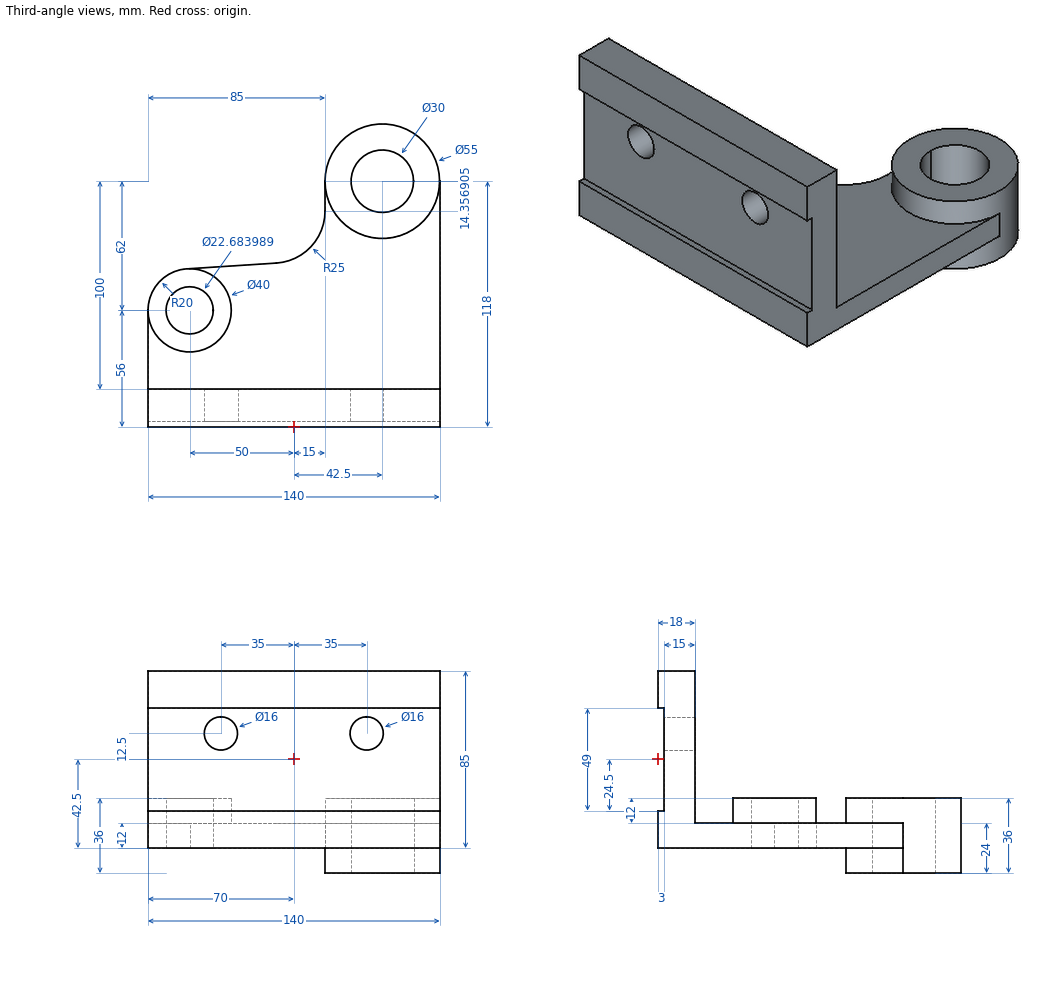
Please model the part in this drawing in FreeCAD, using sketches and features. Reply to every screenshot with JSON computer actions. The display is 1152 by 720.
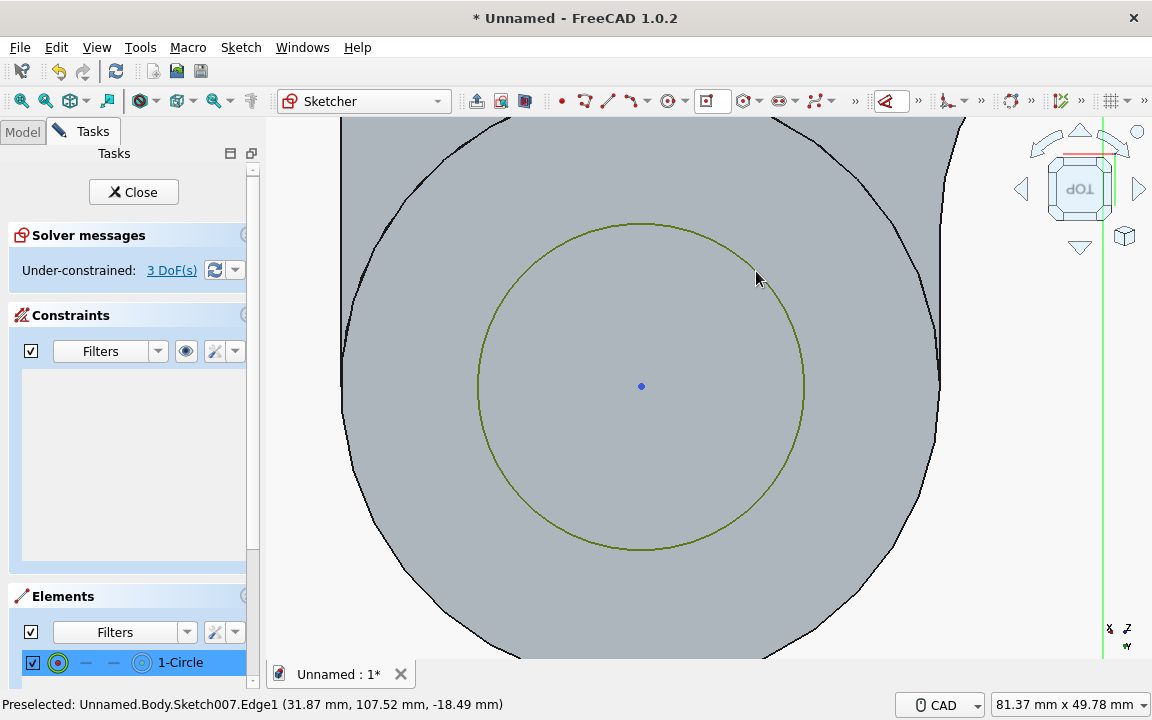
{"action": "left_click", "coordinate": [904, 102]}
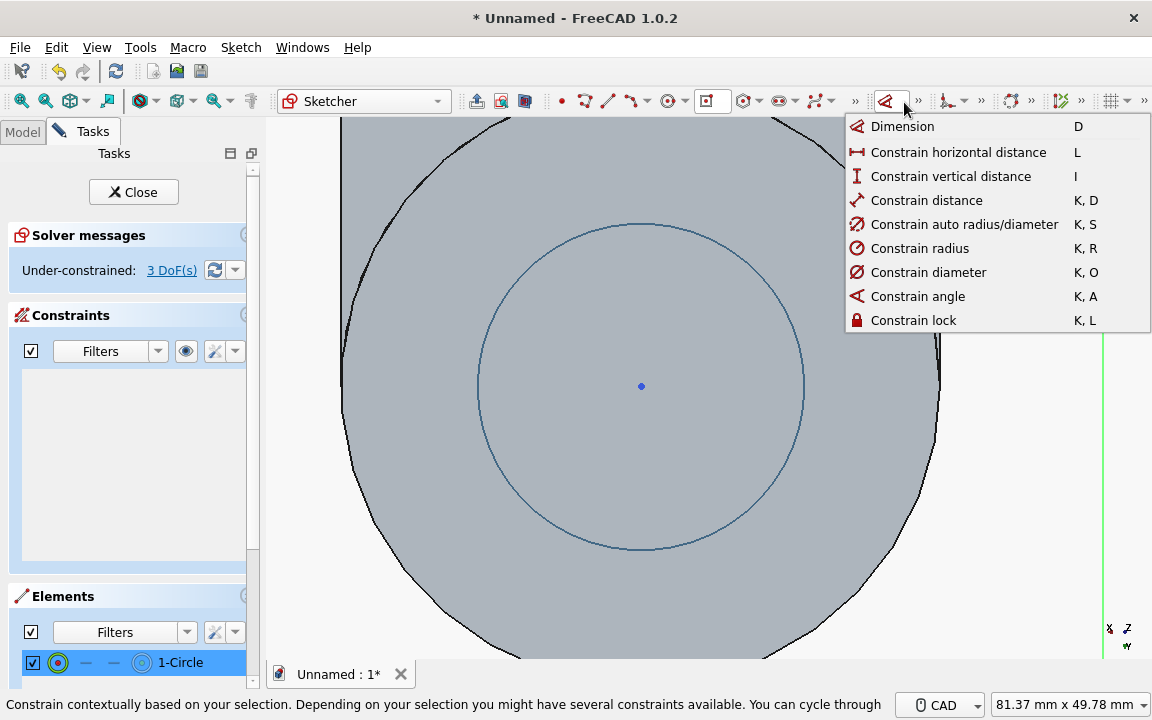
{"action": "left_click", "coordinate": [998, 272]}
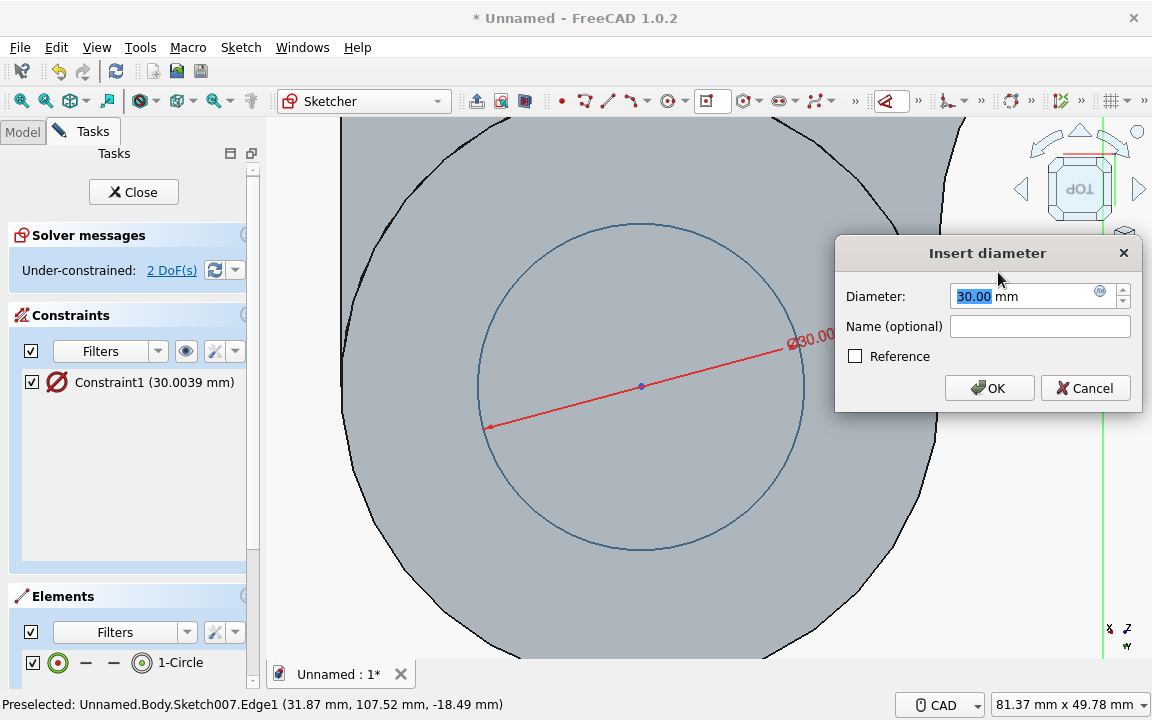
{"action": "type", "text": "30"}
{"action": "key", "text": "Return"}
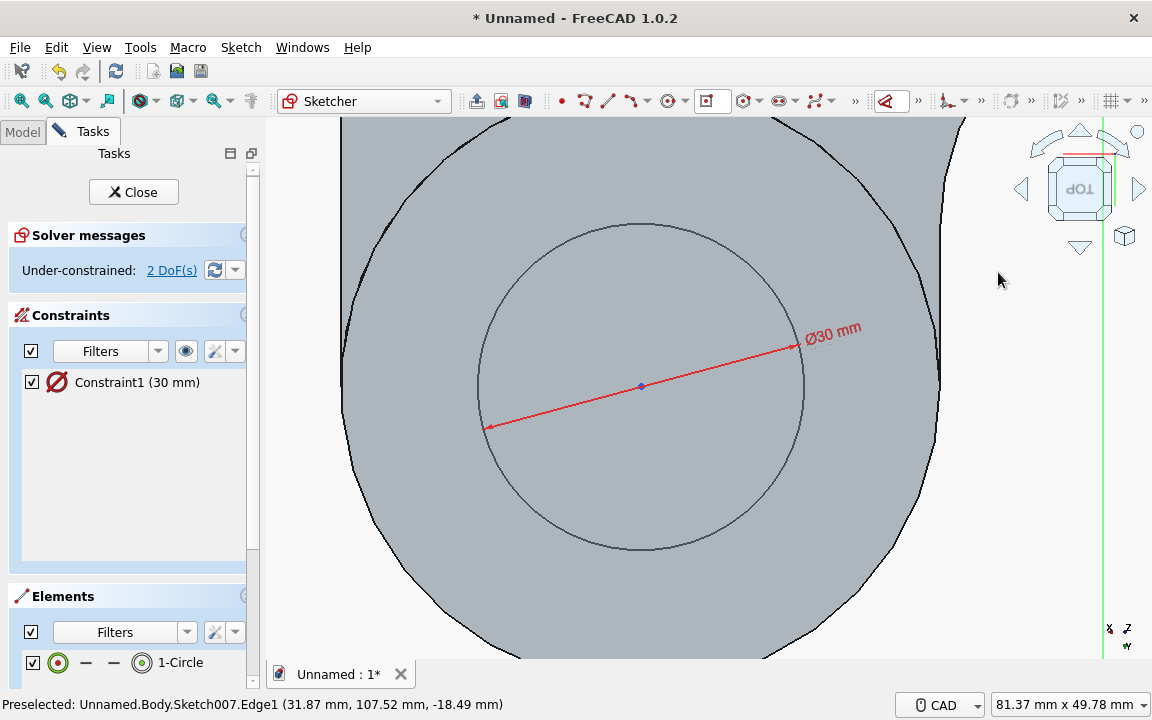
{"action": "left_click", "coordinate": [641, 387]}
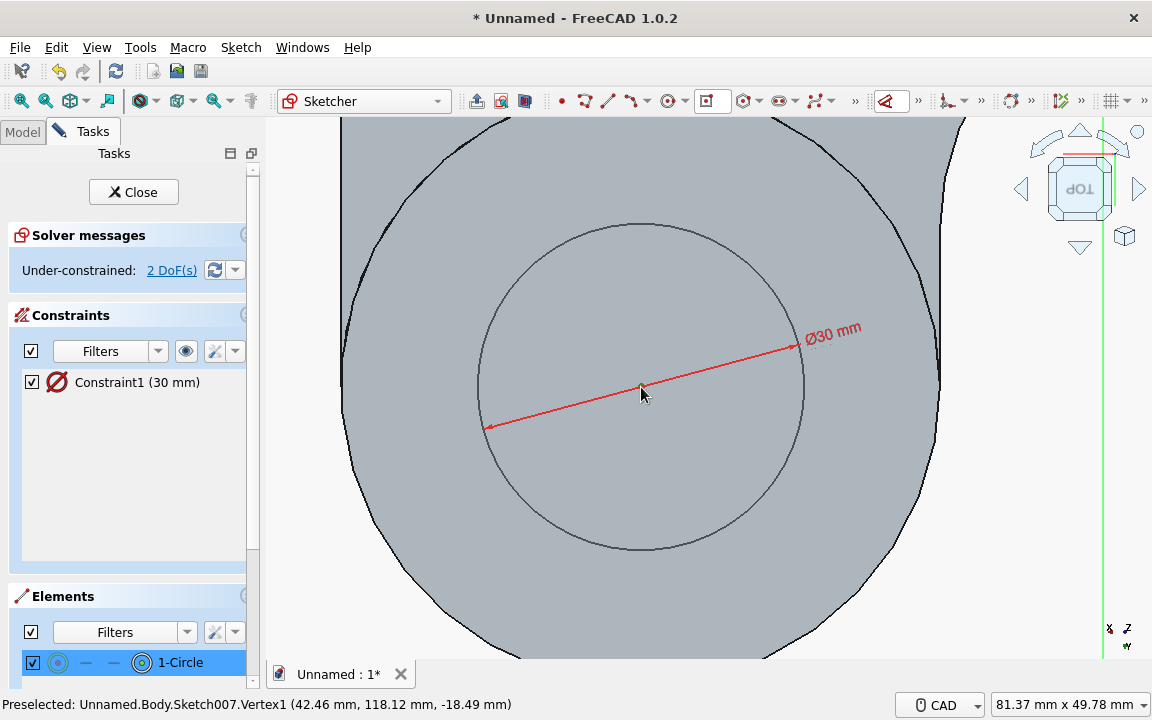
{"action": "left_click", "coordinate": [904, 102]}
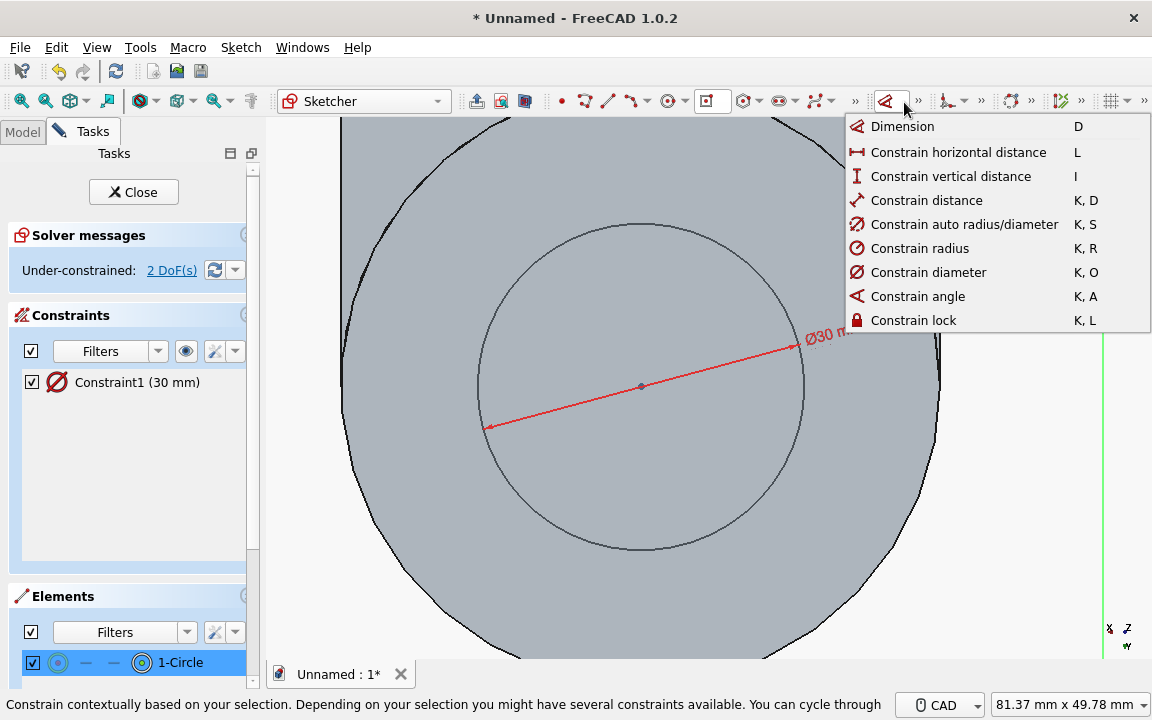
{"action": "left_click", "coordinate": [998, 176]}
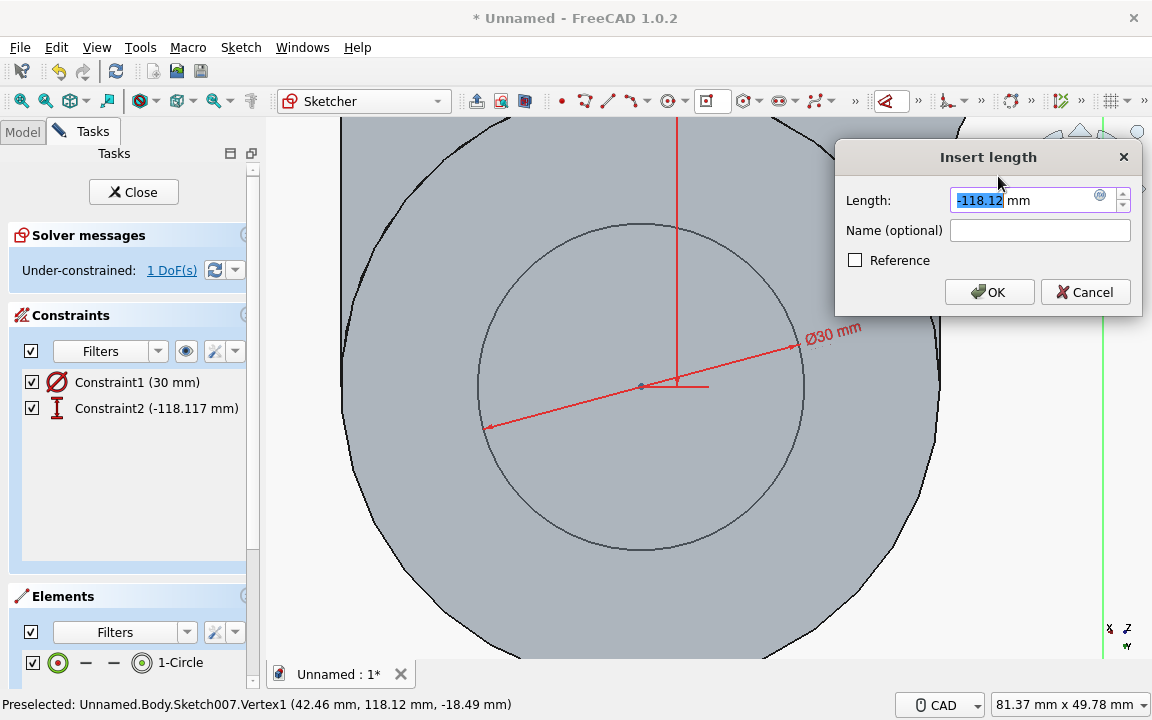
{"action": "type", "text": "-118"}
{"action": "key", "text": "Return"}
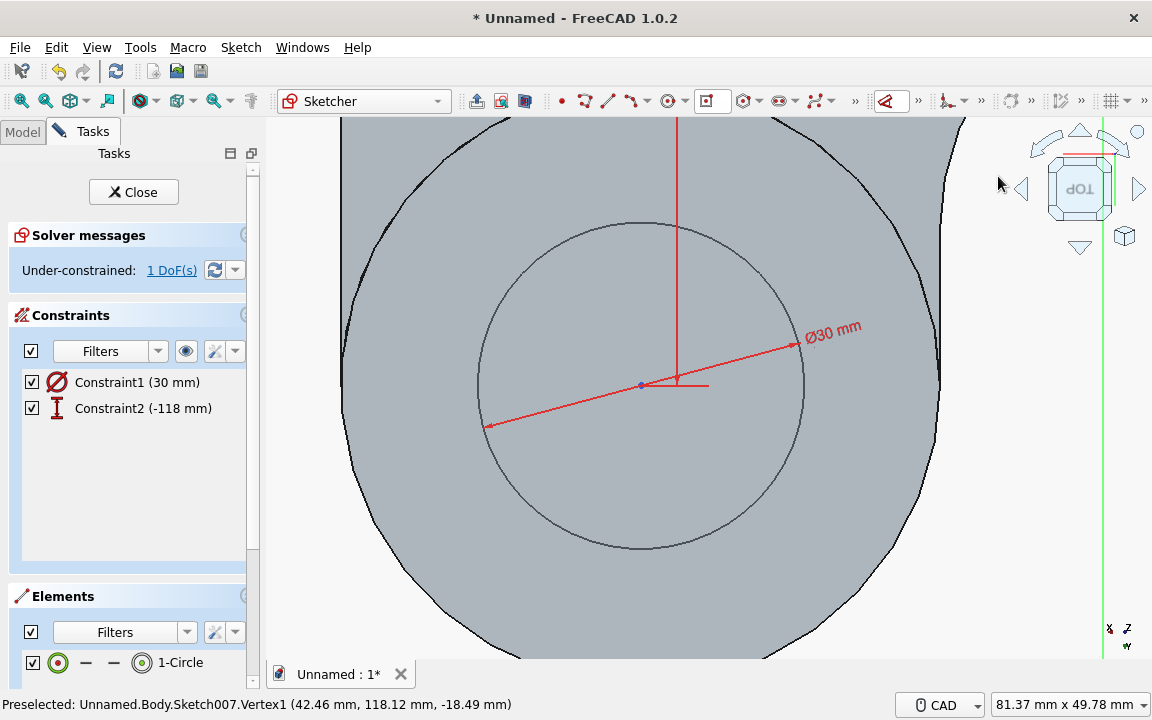
{"action": "left_click", "coordinate": [641, 386]}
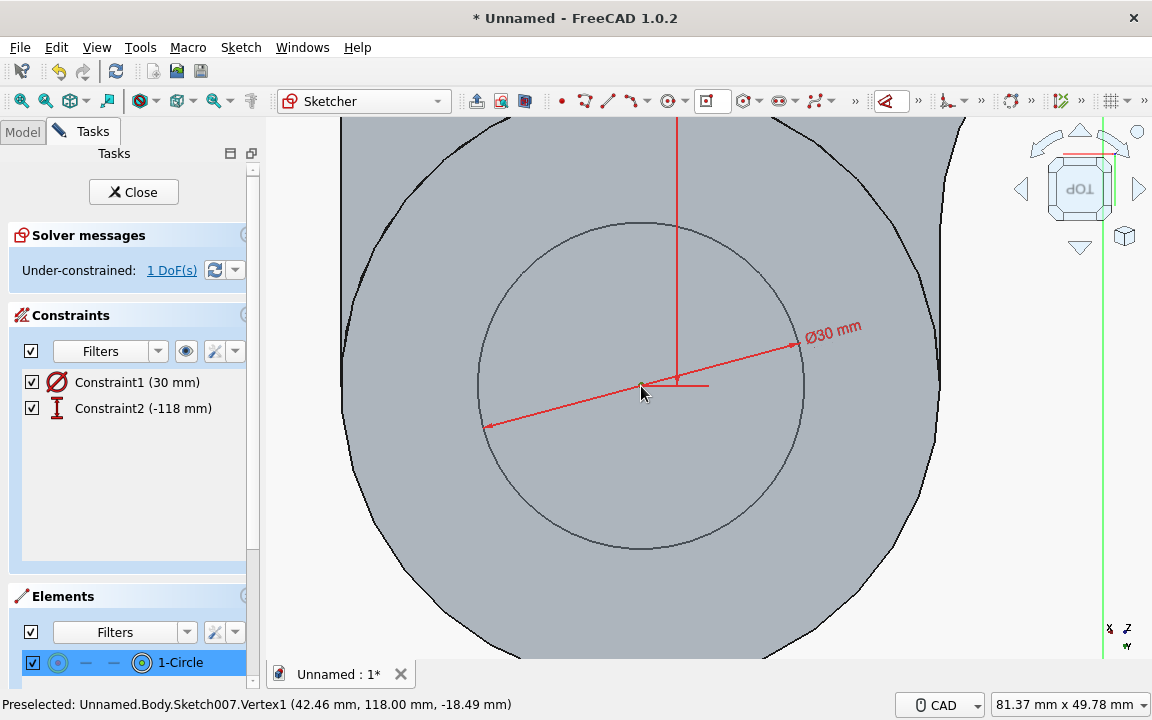
{"action": "key", "text": "l"}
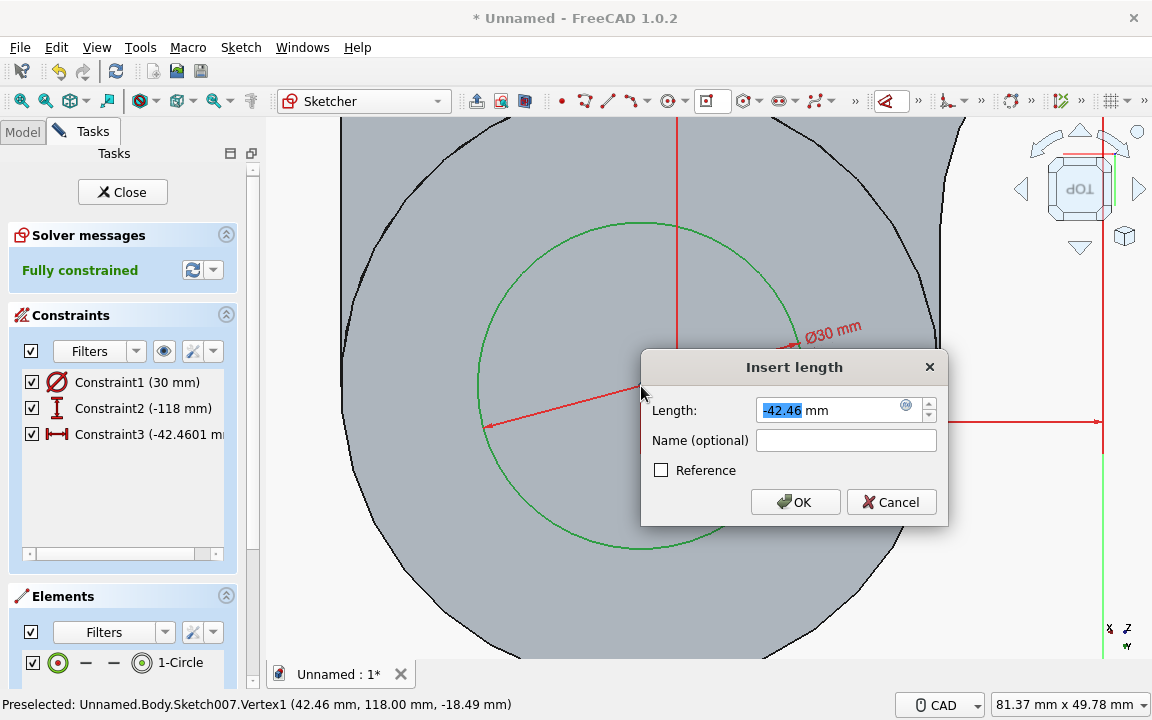
{"action": "type", "text": "-42.5"}
{"action": "key", "text": "Return"}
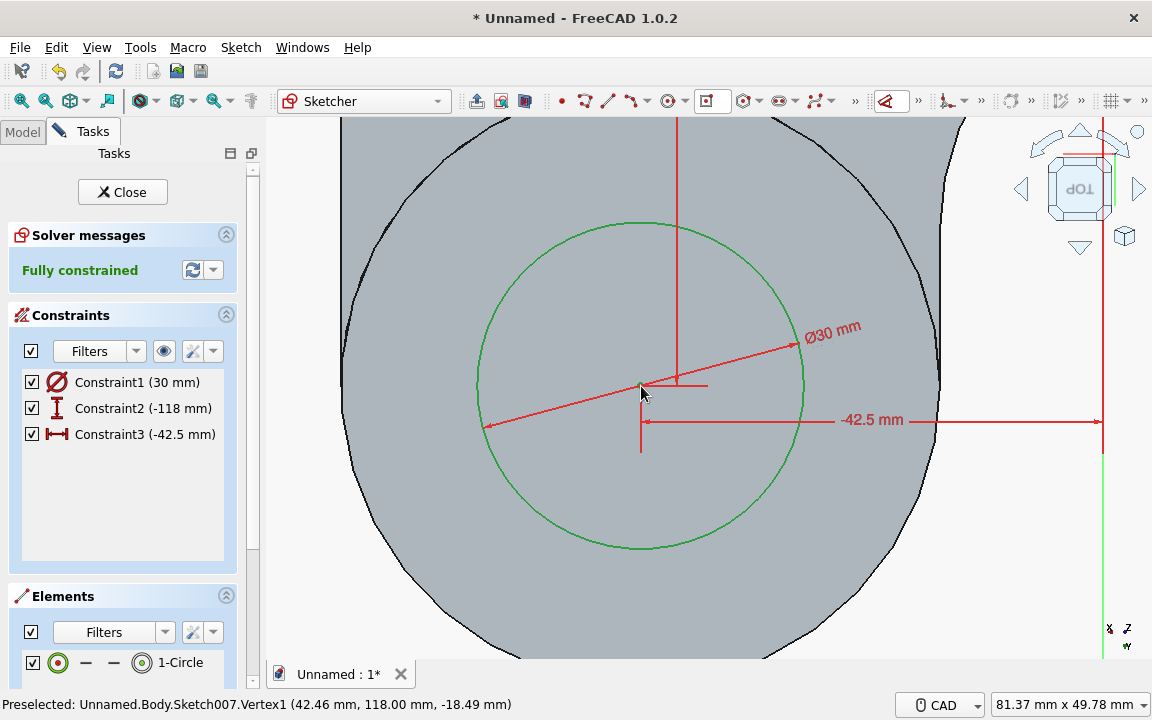
{"action": "left_click", "coordinate": [123, 192]}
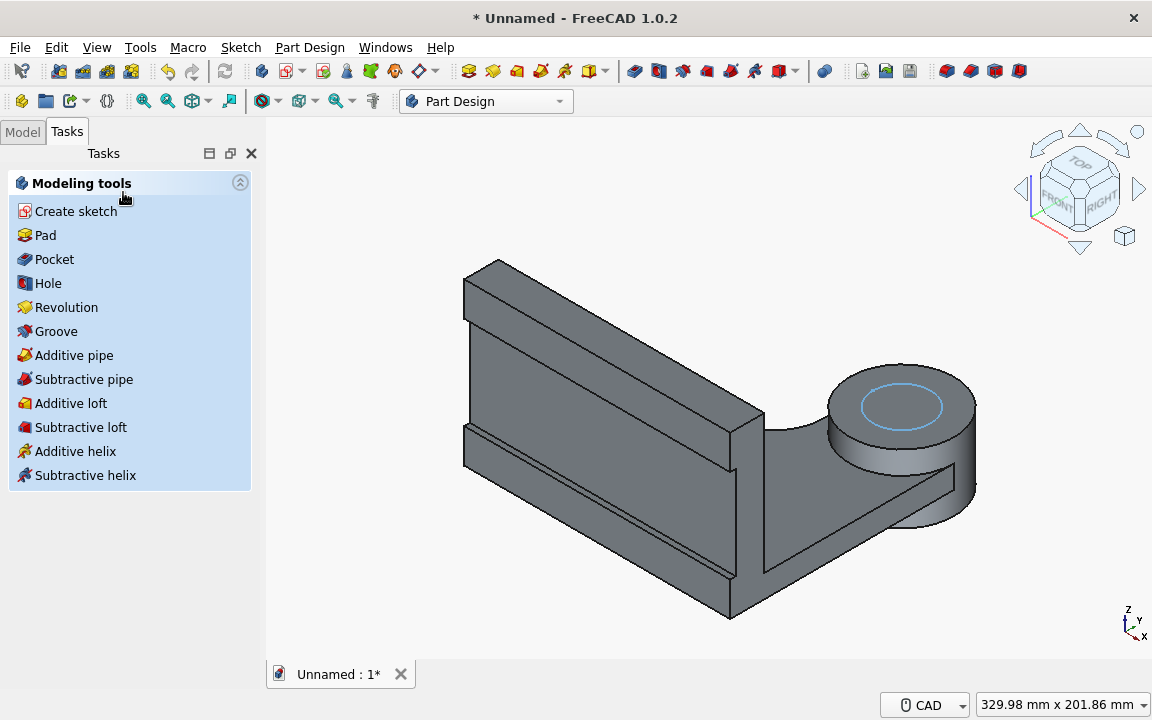
{"action": "left_click", "coordinate": [636, 72]}